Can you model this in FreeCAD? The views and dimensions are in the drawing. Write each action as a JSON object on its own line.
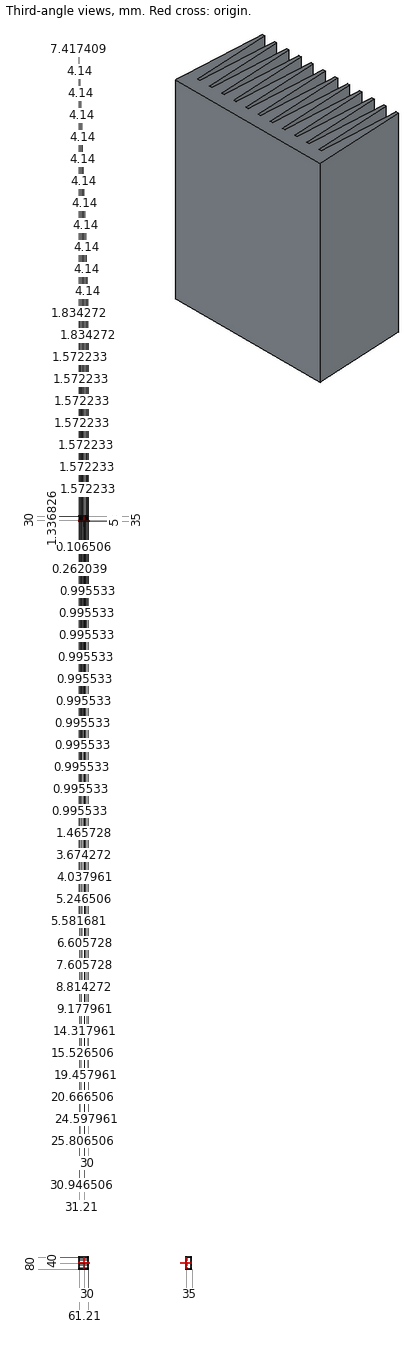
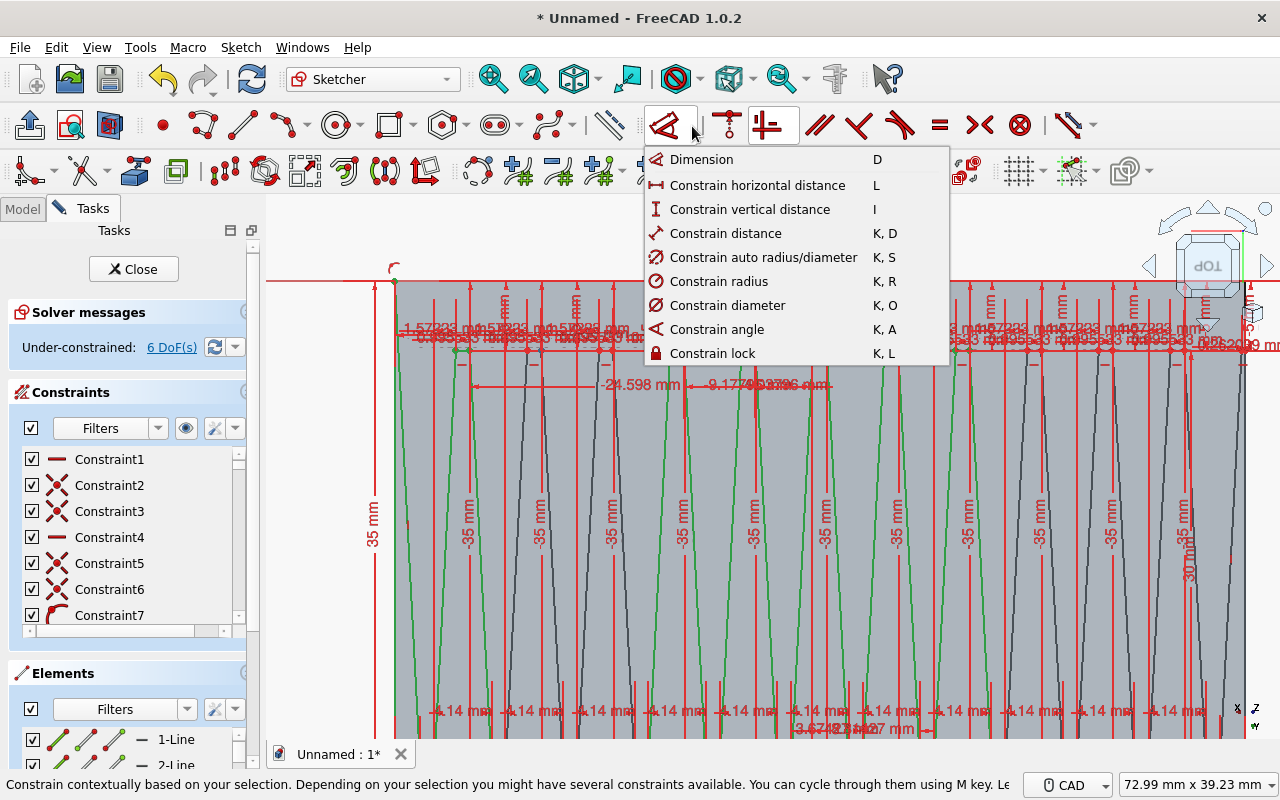
{"action": "left_click", "coordinate": [797, 185]}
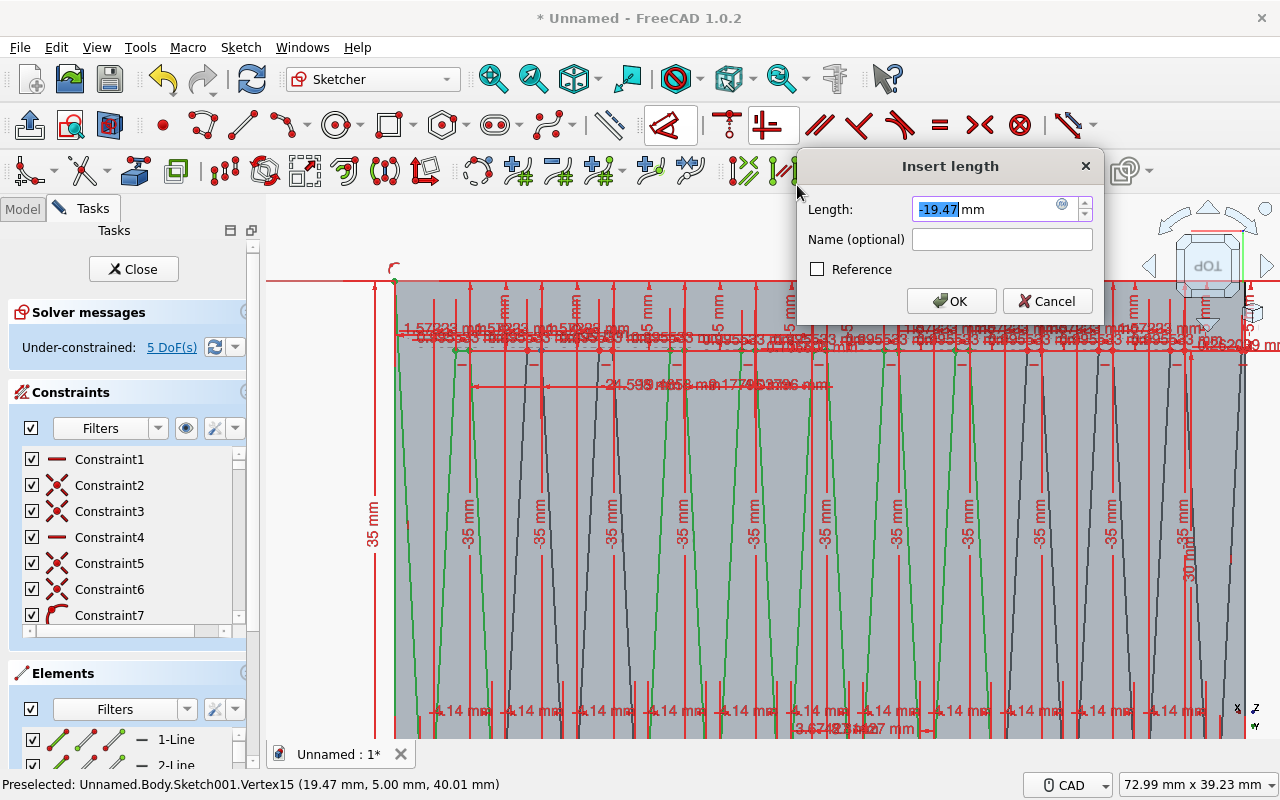
{"action": "type", "text": "-19.457961"}
{"action": "key", "text": "Return"}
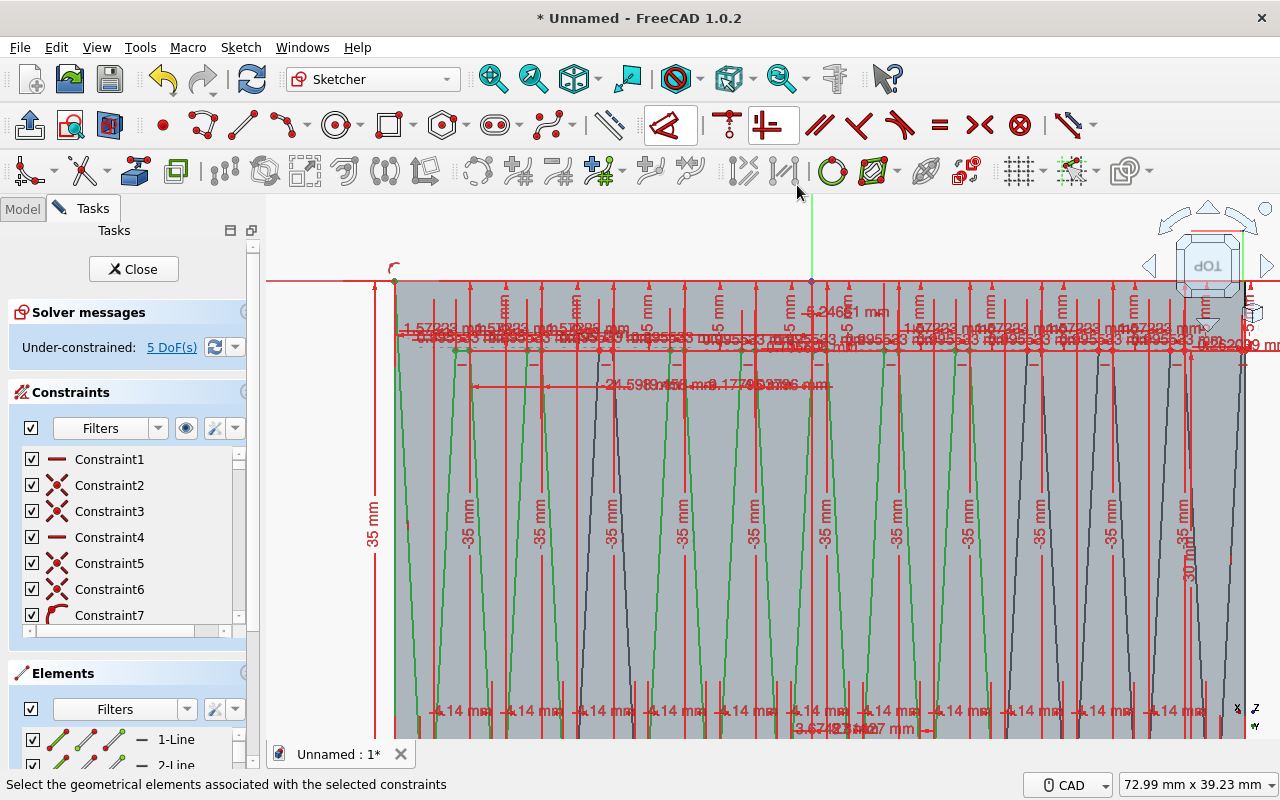
{"action": "left_click", "coordinate": [613, 351]}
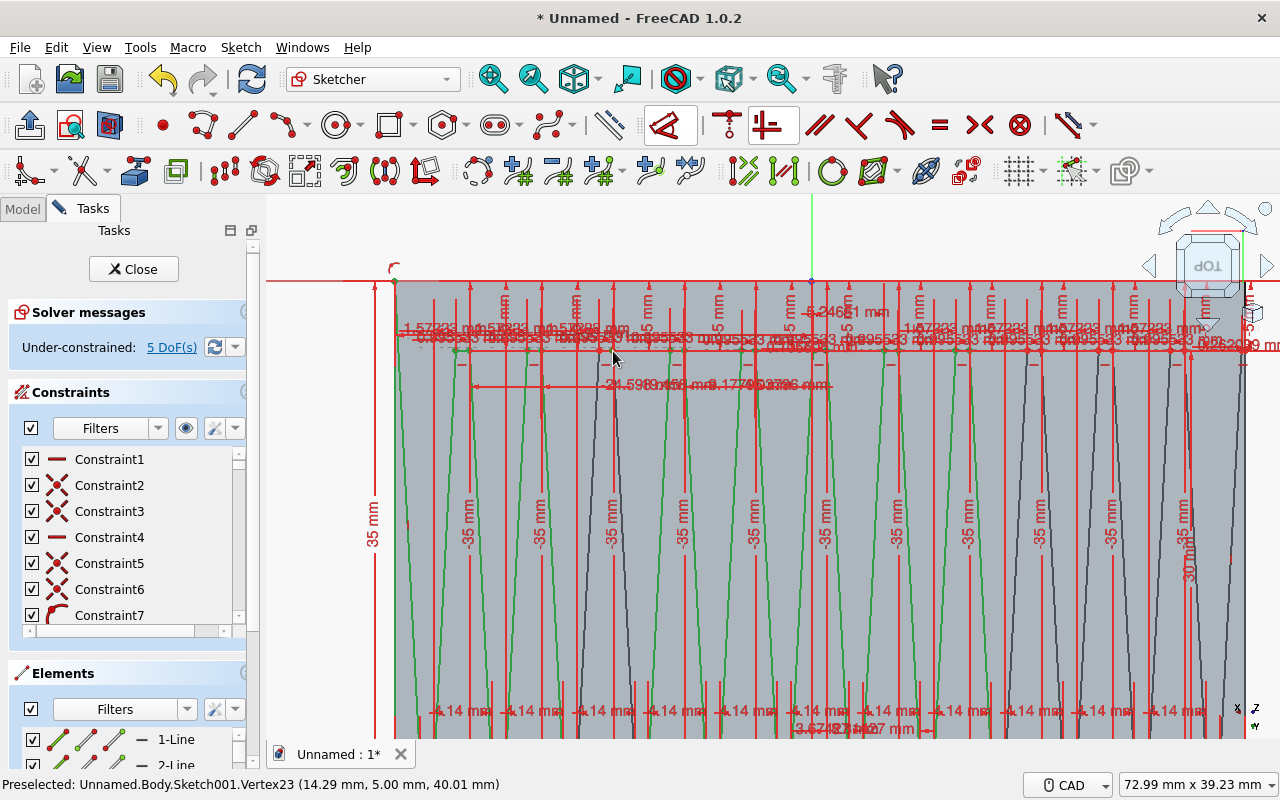
{"action": "key", "text": "l"}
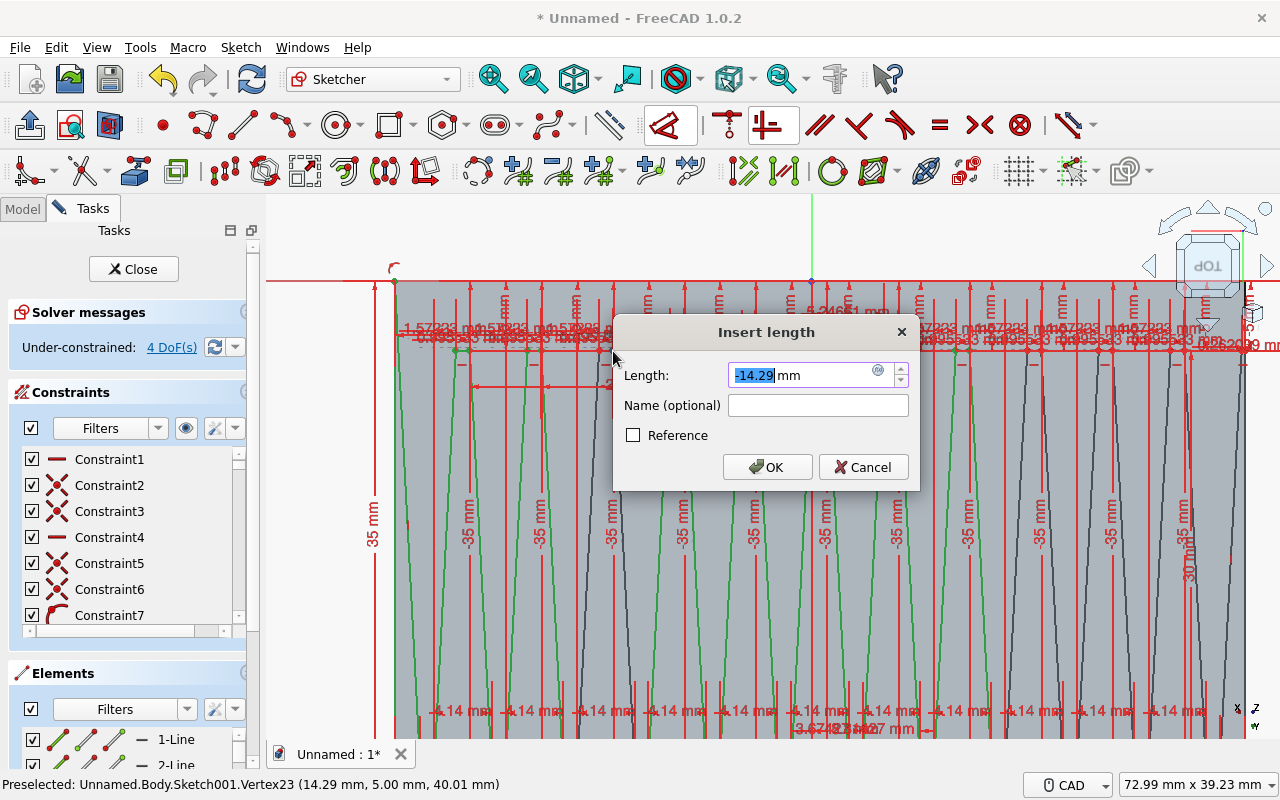
{"action": "type", "text": "-14.317961"}
{"action": "key", "text": "Return"}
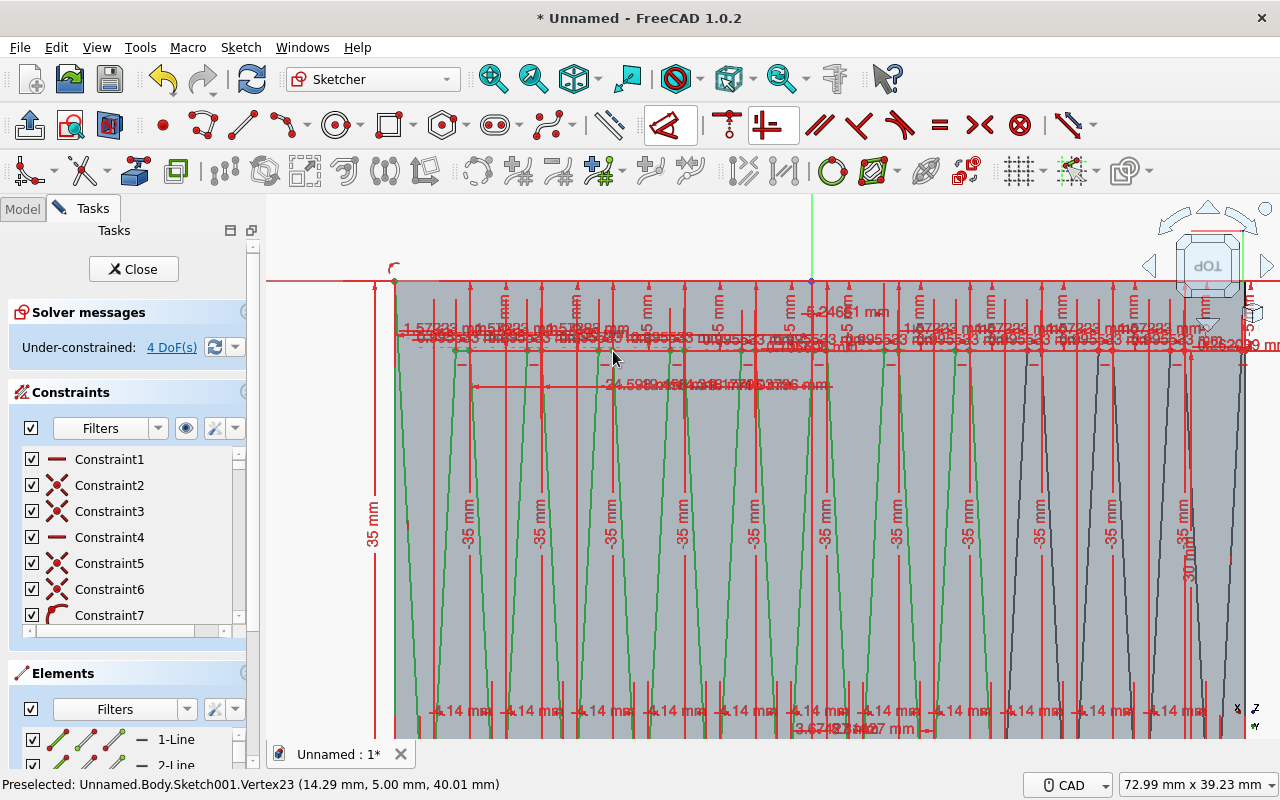
{"action": "left_click", "coordinate": [1027, 351]}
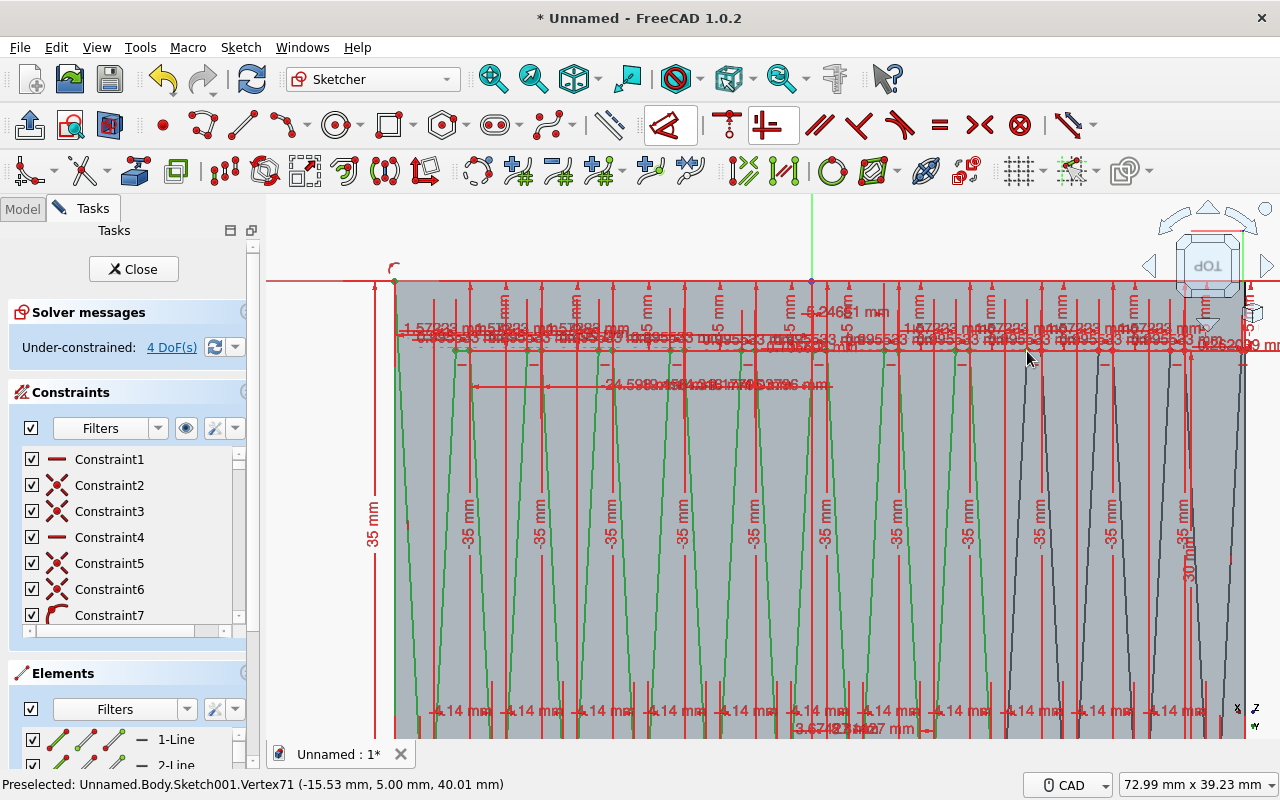
{"action": "key", "text": "l"}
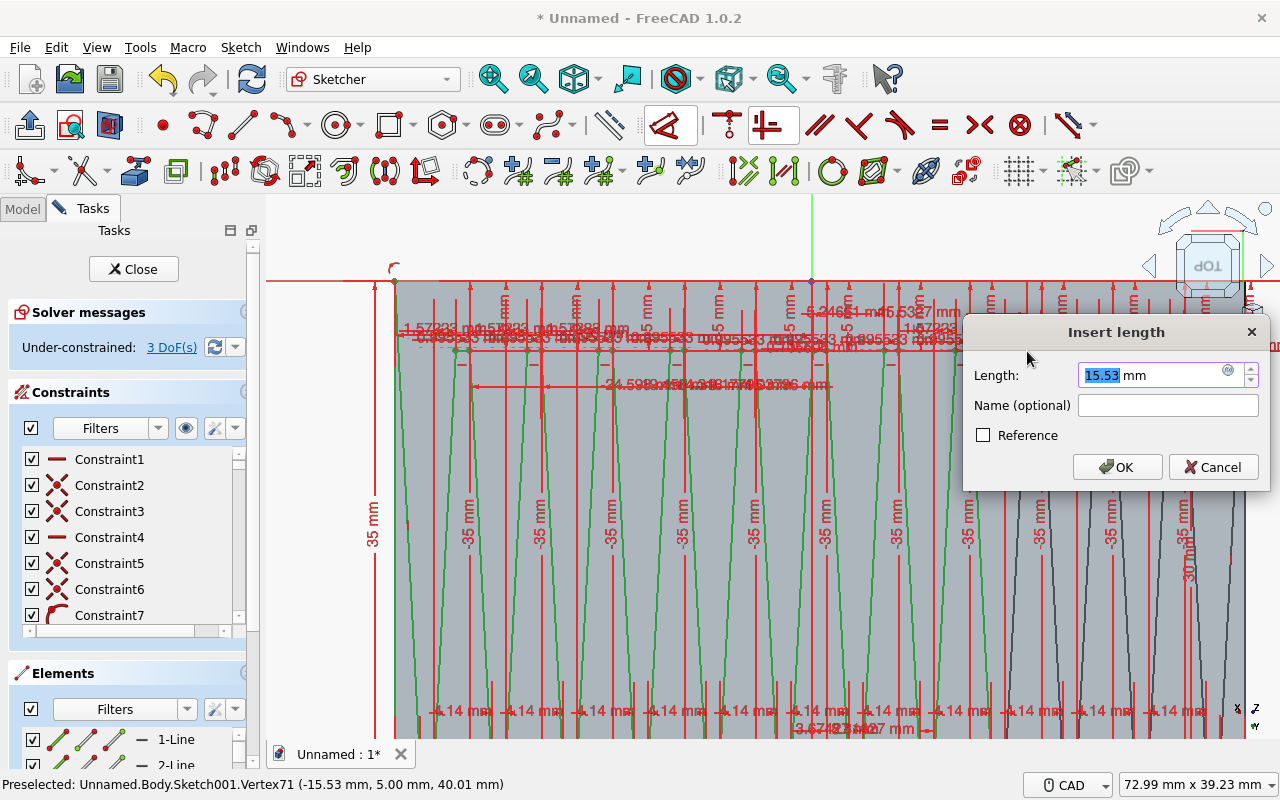
{"action": "type", "text": "15.526506"}
{"action": "key", "text": "Return"}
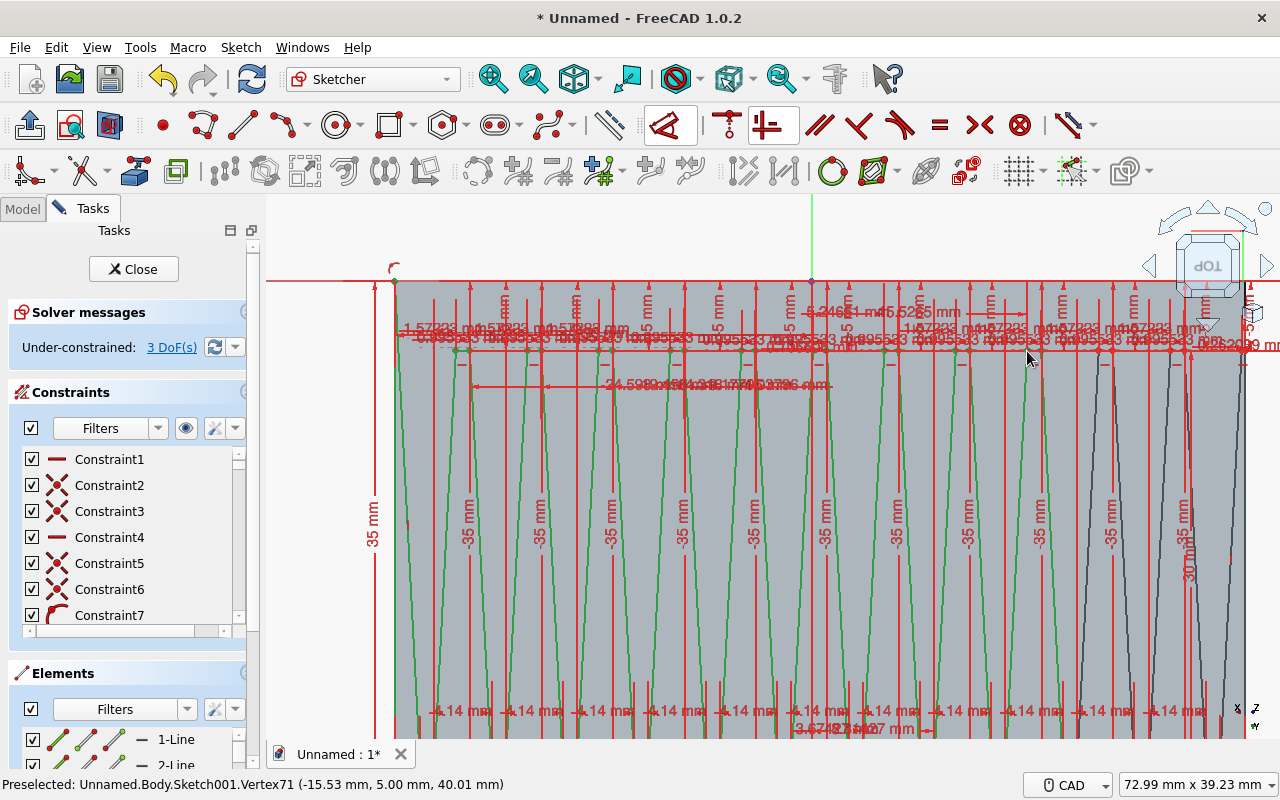
{"action": "left_click", "coordinate": [1099, 351]}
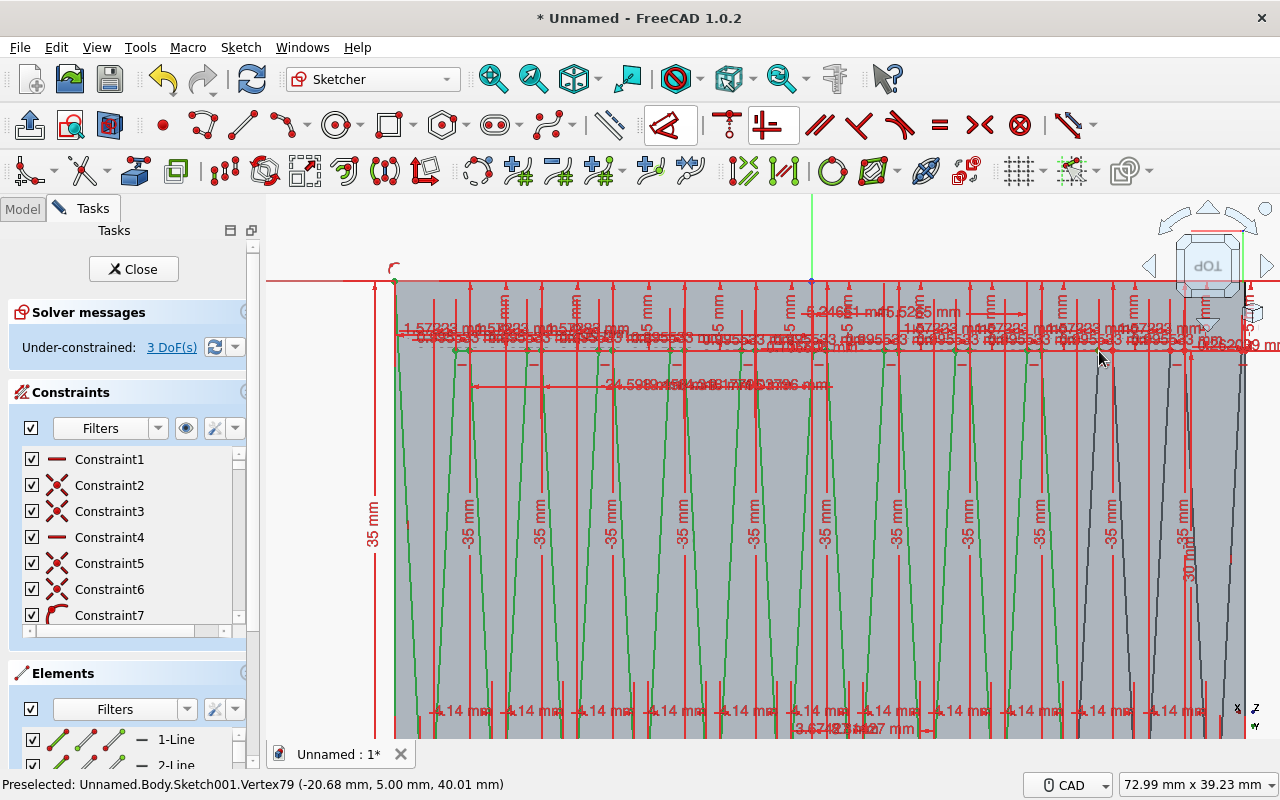
{"action": "left_click", "coordinate": [692, 126]}